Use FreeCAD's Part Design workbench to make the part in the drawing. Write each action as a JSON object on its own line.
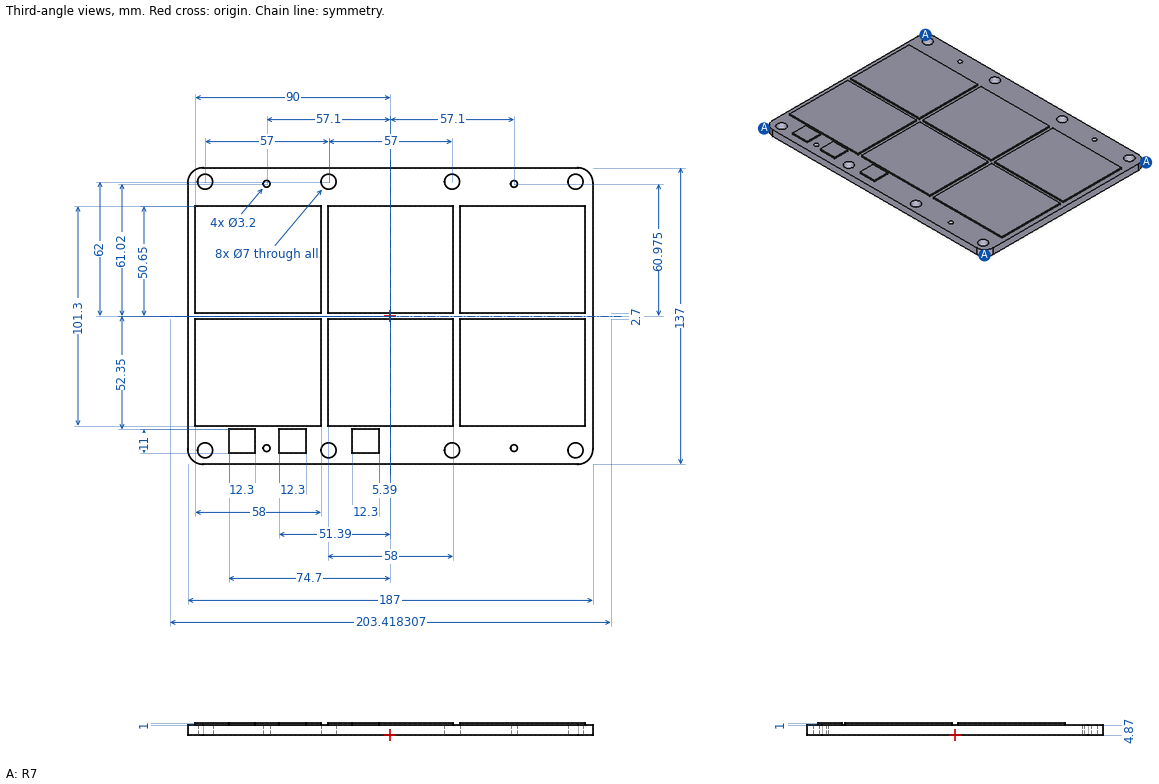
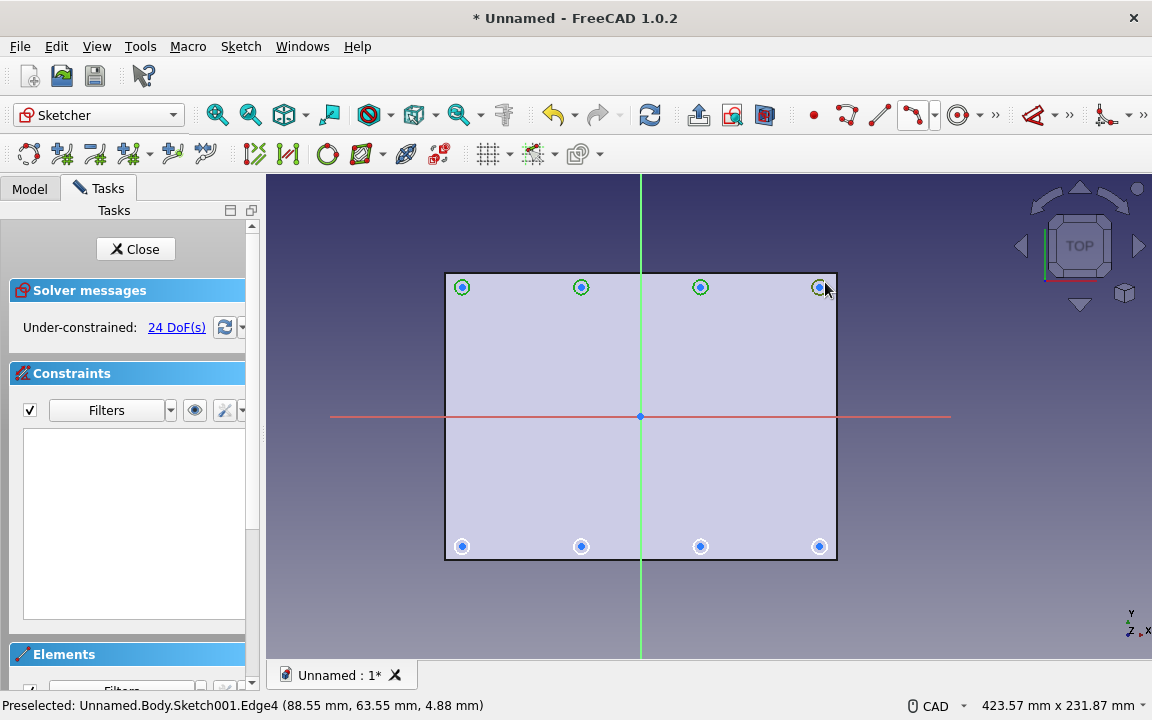
{"action": "scroll", "coordinate": [825, 541], "scroll_direction": "up", "scroll_amount": 4}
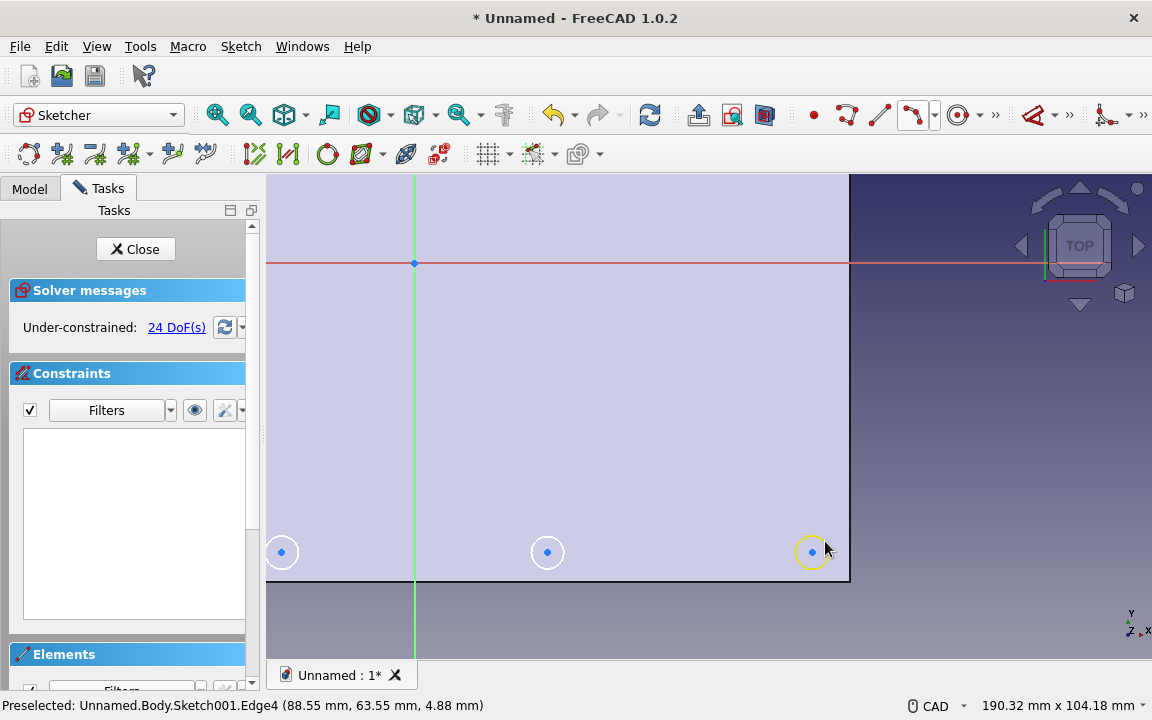
{"action": "left_click", "coordinate": [824, 541]}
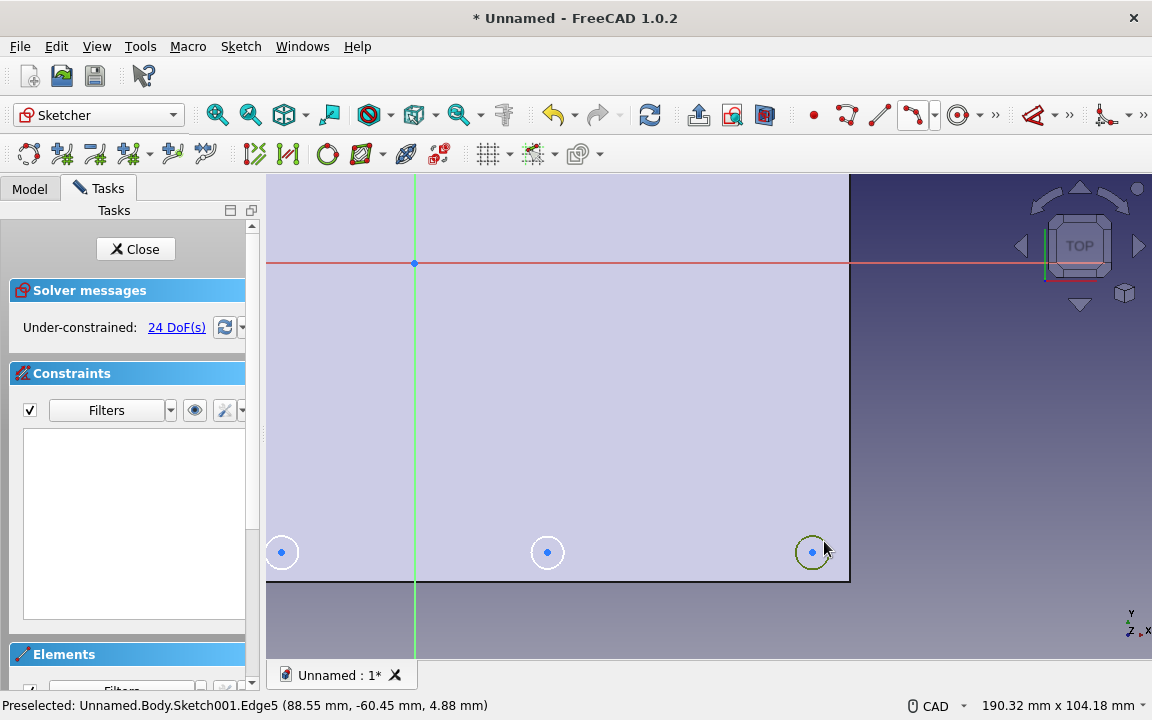
{"action": "left_click", "coordinate": [559, 541]}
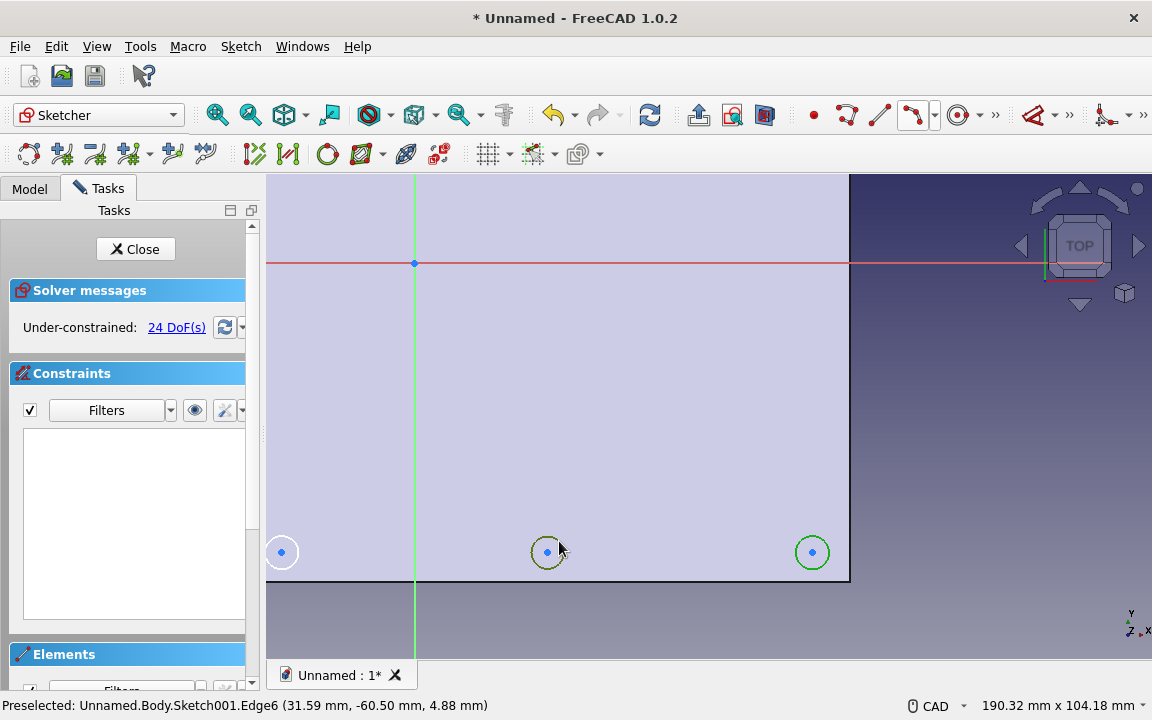
{"action": "scroll", "coordinate": [825, 541], "scroll_direction": "down", "scroll_amount": 4}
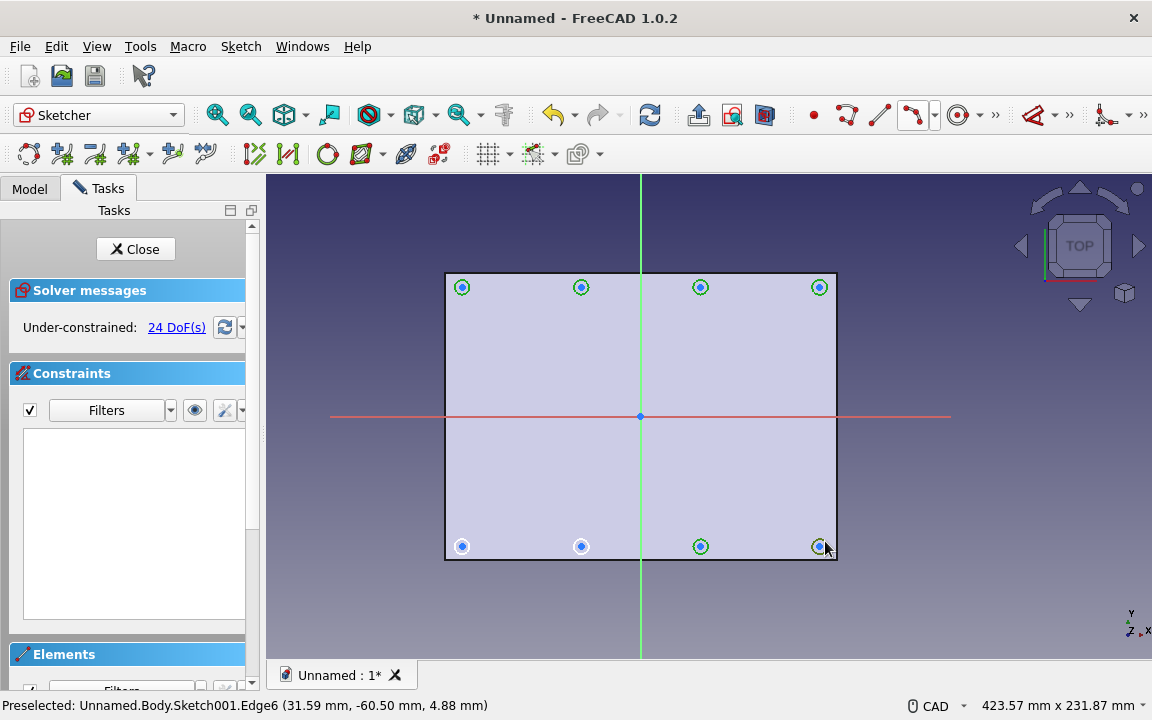
{"action": "scroll", "coordinate": [467, 541], "scroll_direction": "up", "scroll_amount": 4}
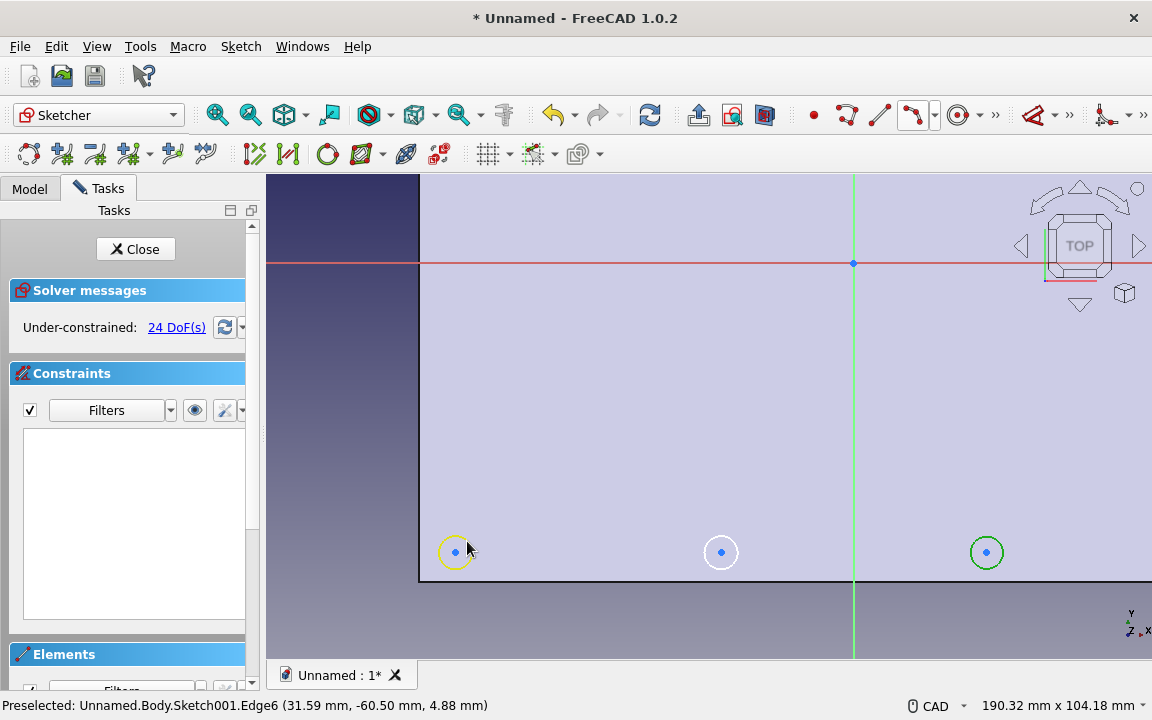
{"action": "left_click", "coordinate": [467, 541]}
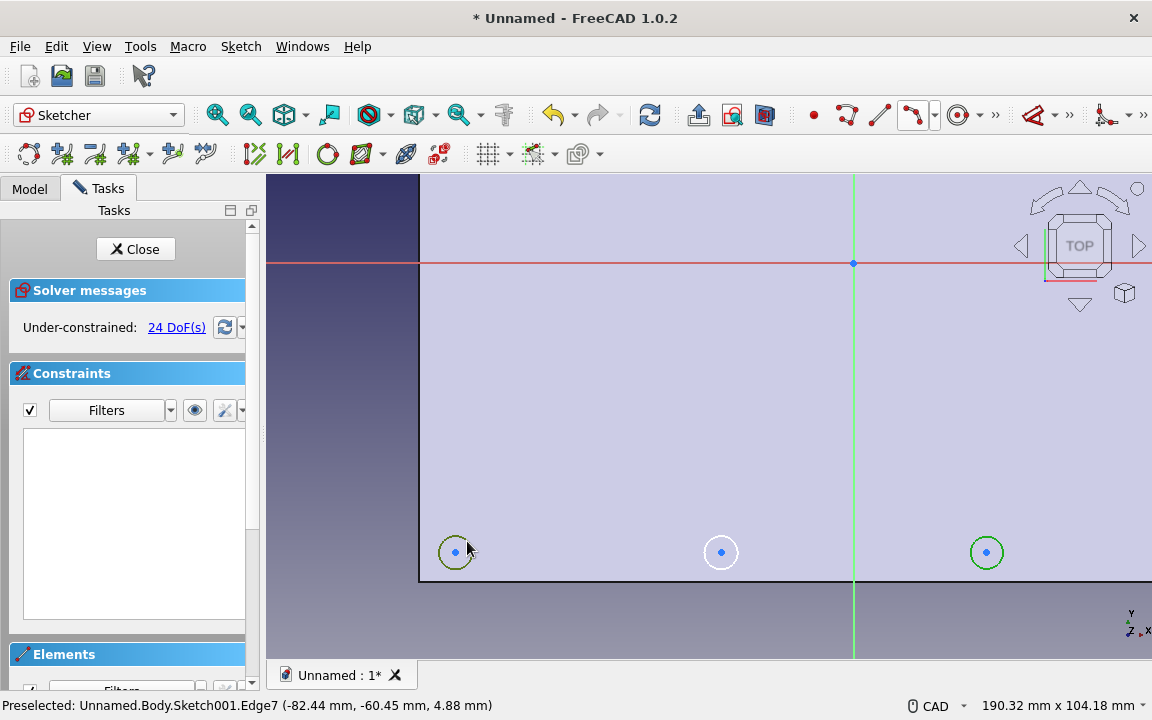
{"action": "left_click", "coordinate": [733, 541]}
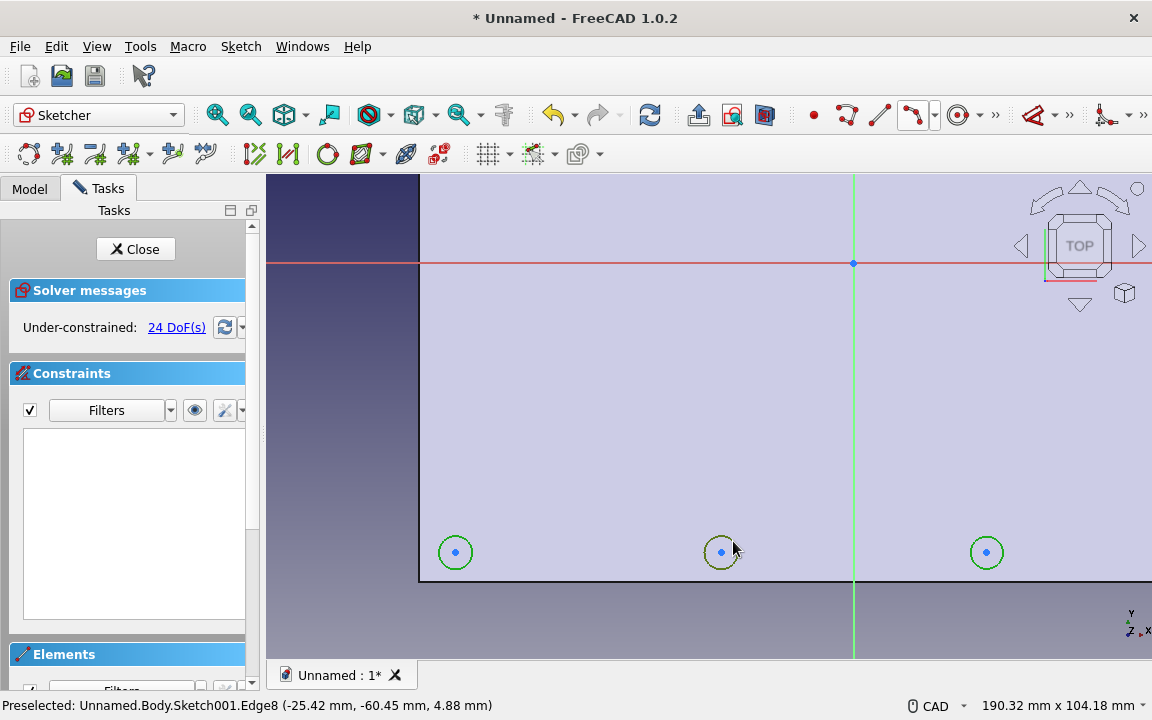
{"action": "key", "text": "e"}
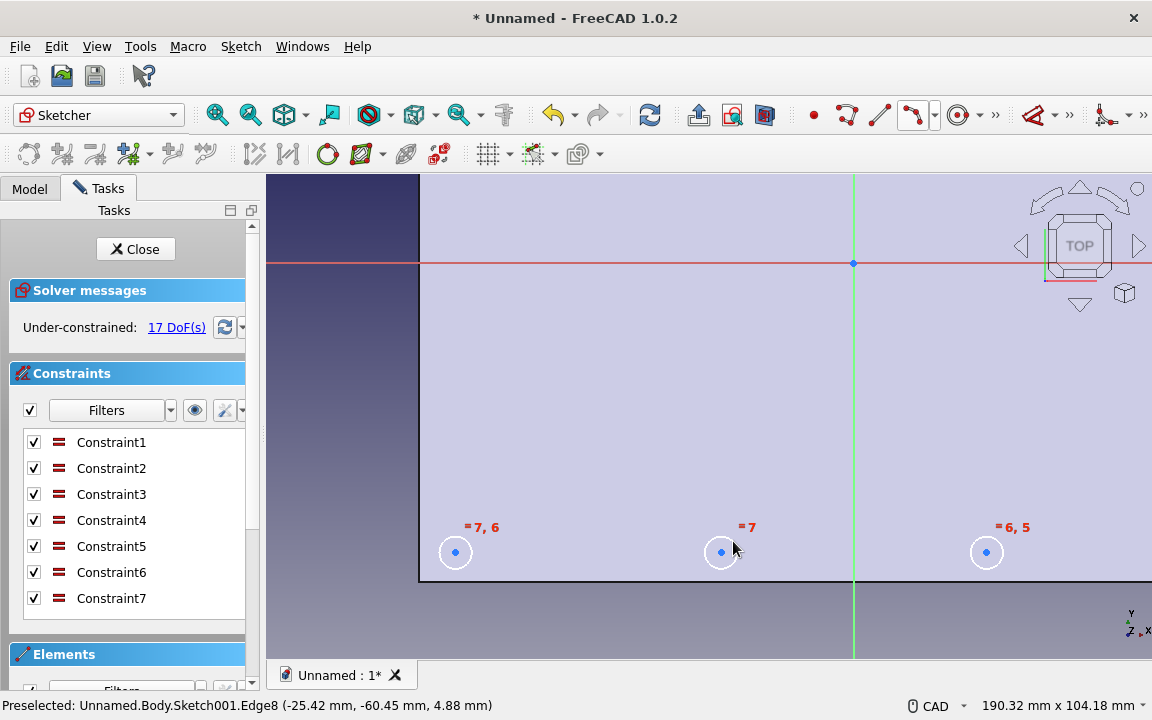
{"action": "scroll", "coordinate": [466, 541], "scroll_direction": "down", "scroll_amount": 4}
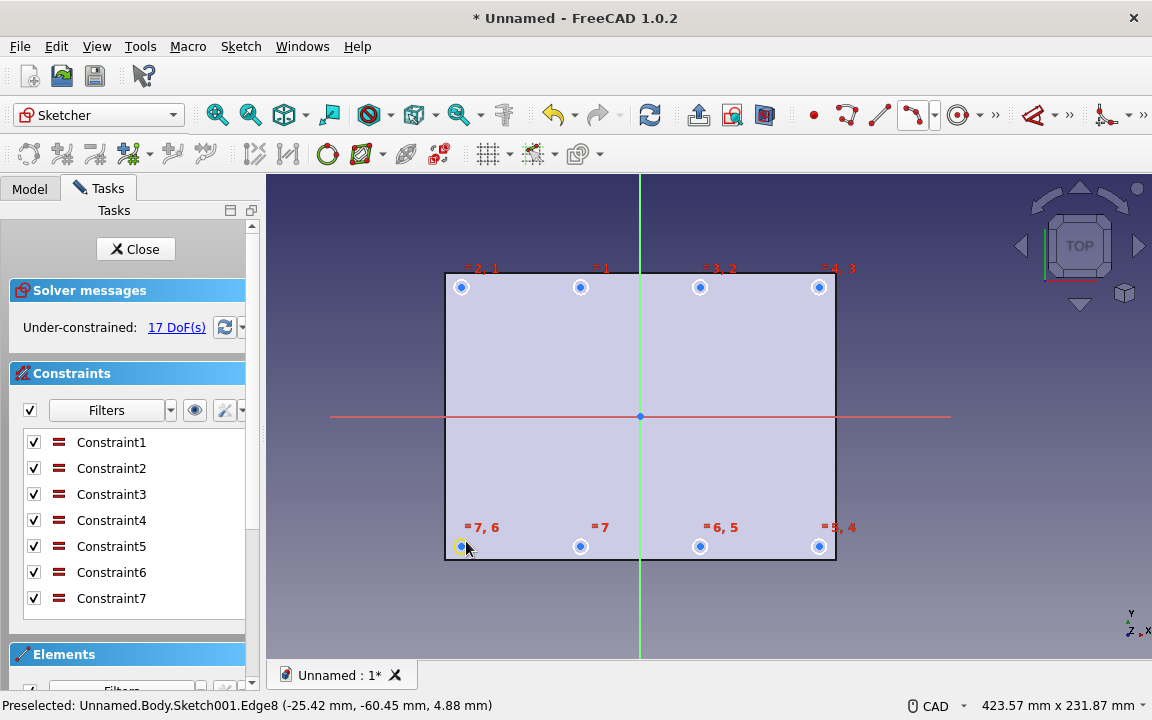
{"action": "left_click", "coordinate": [581, 287]}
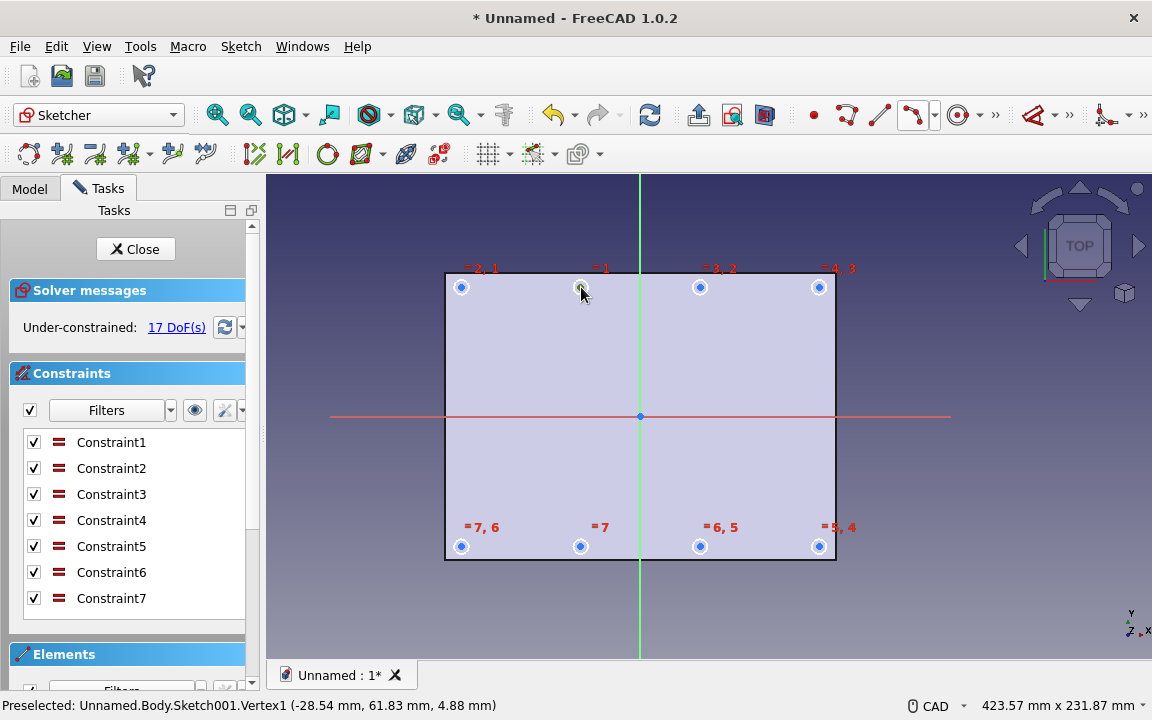
{"action": "left_click", "coordinate": [700, 287]}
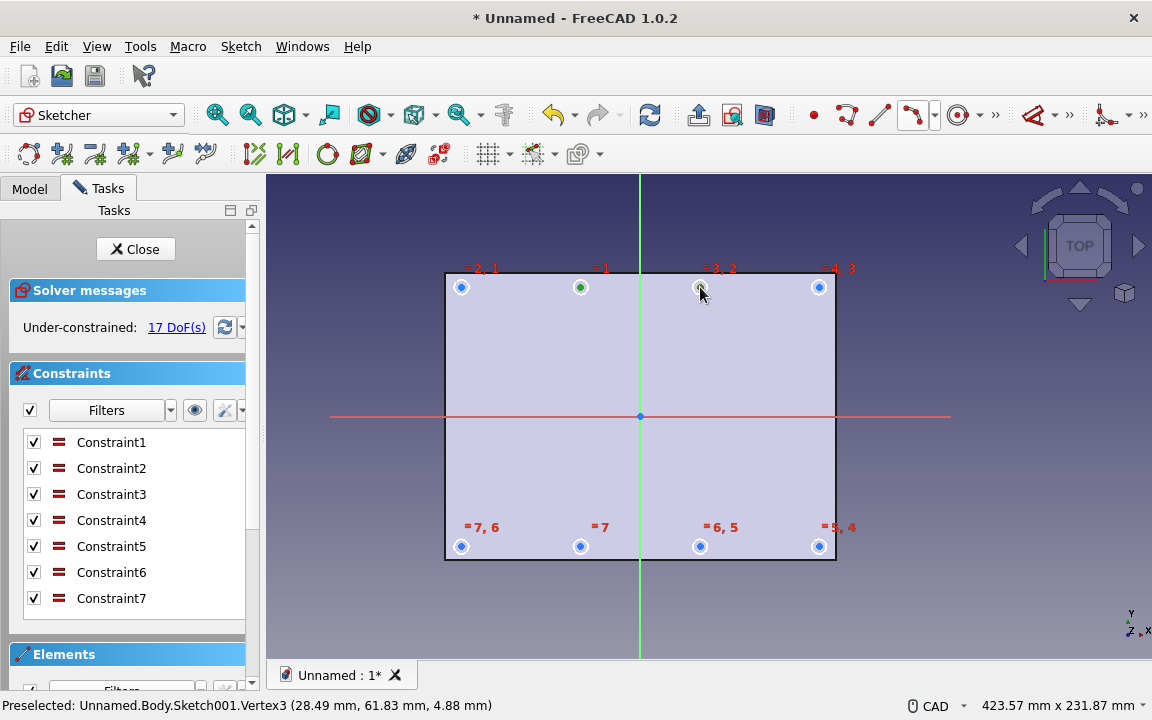
{"action": "left_click", "coordinate": [640, 600]}